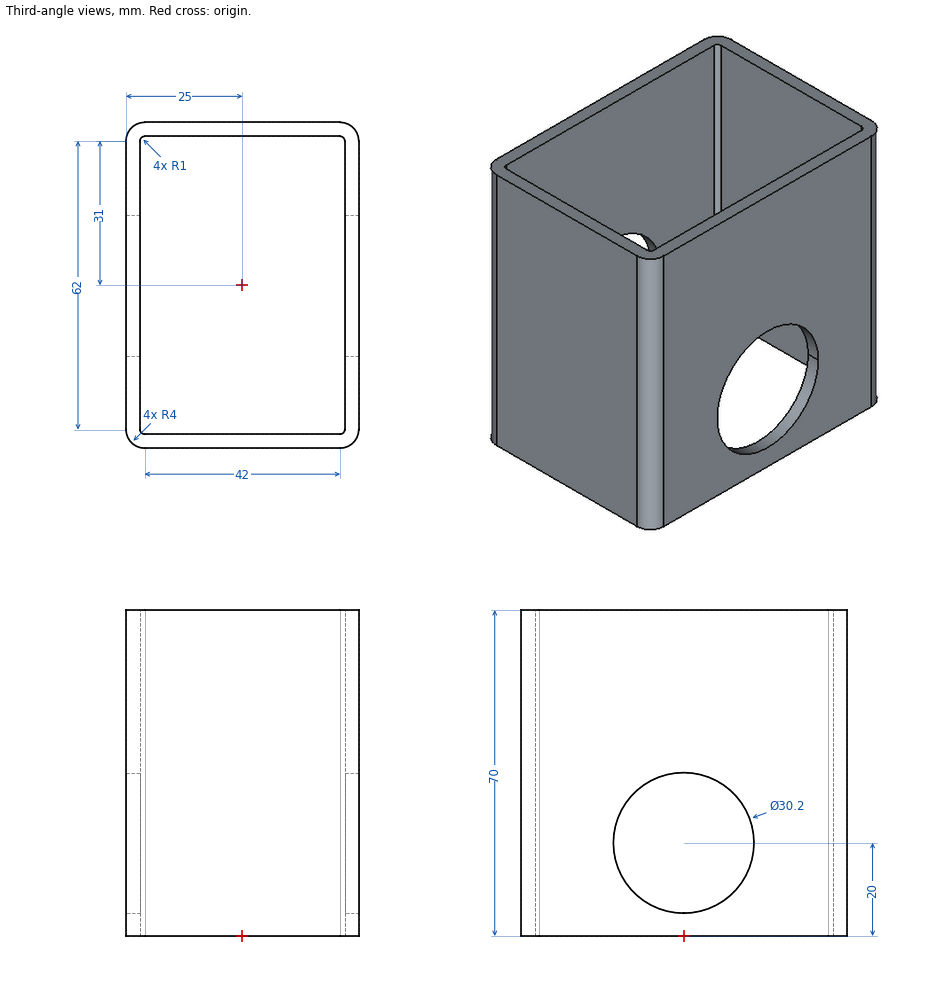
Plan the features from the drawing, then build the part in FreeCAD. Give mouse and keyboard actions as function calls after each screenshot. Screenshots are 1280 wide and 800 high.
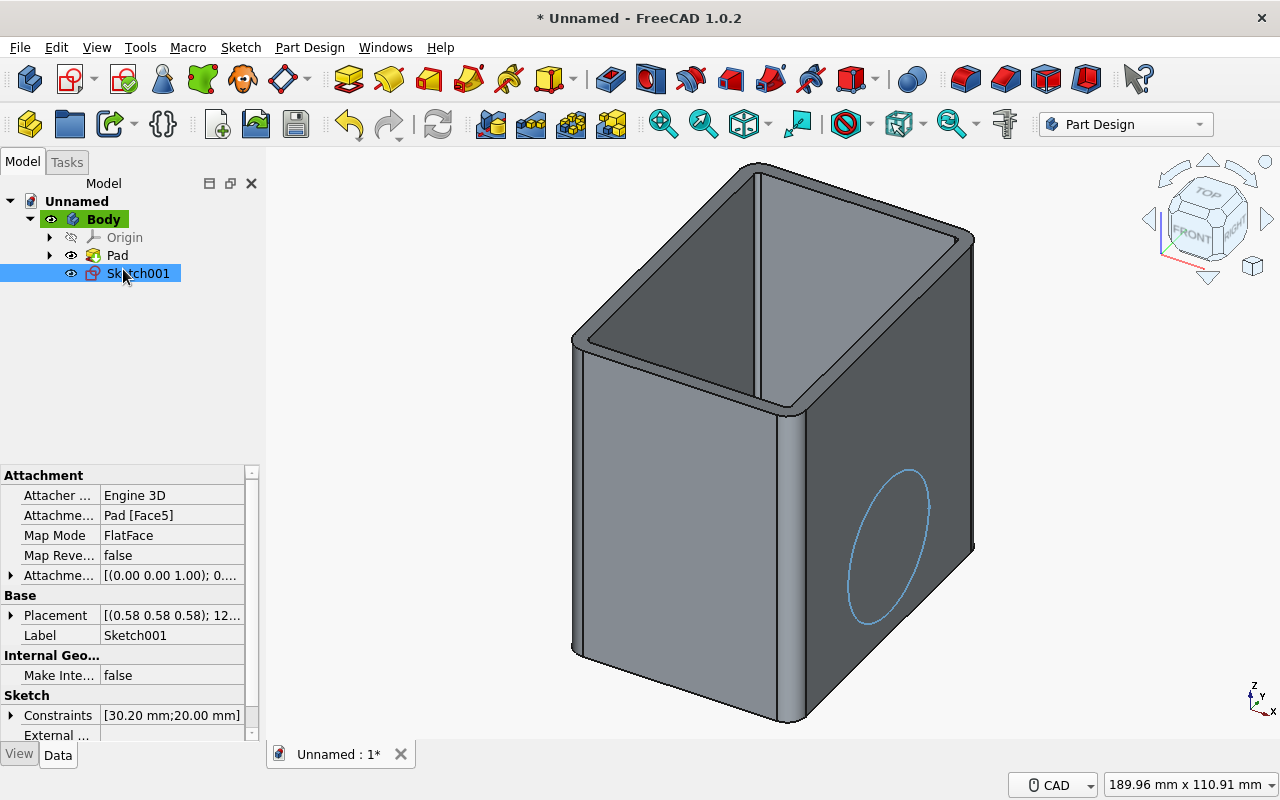
click(612, 80)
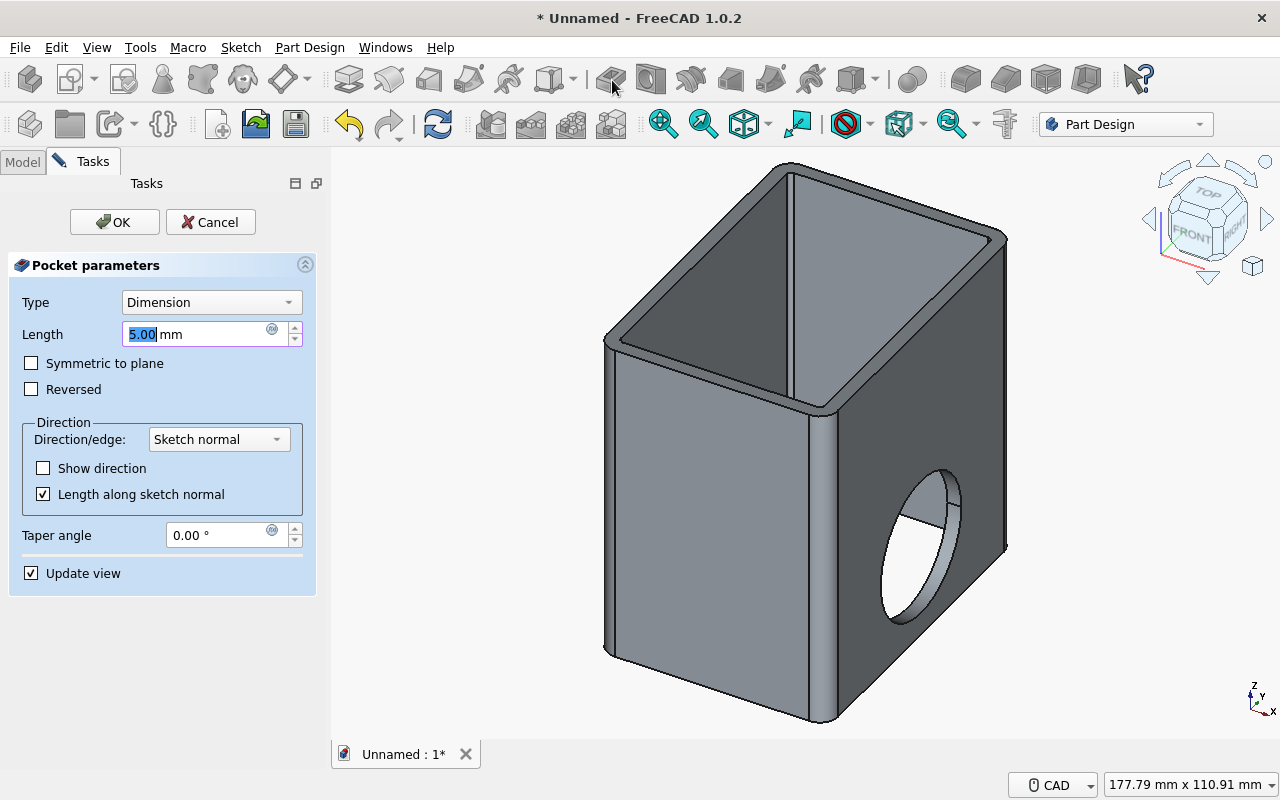
click(212, 302)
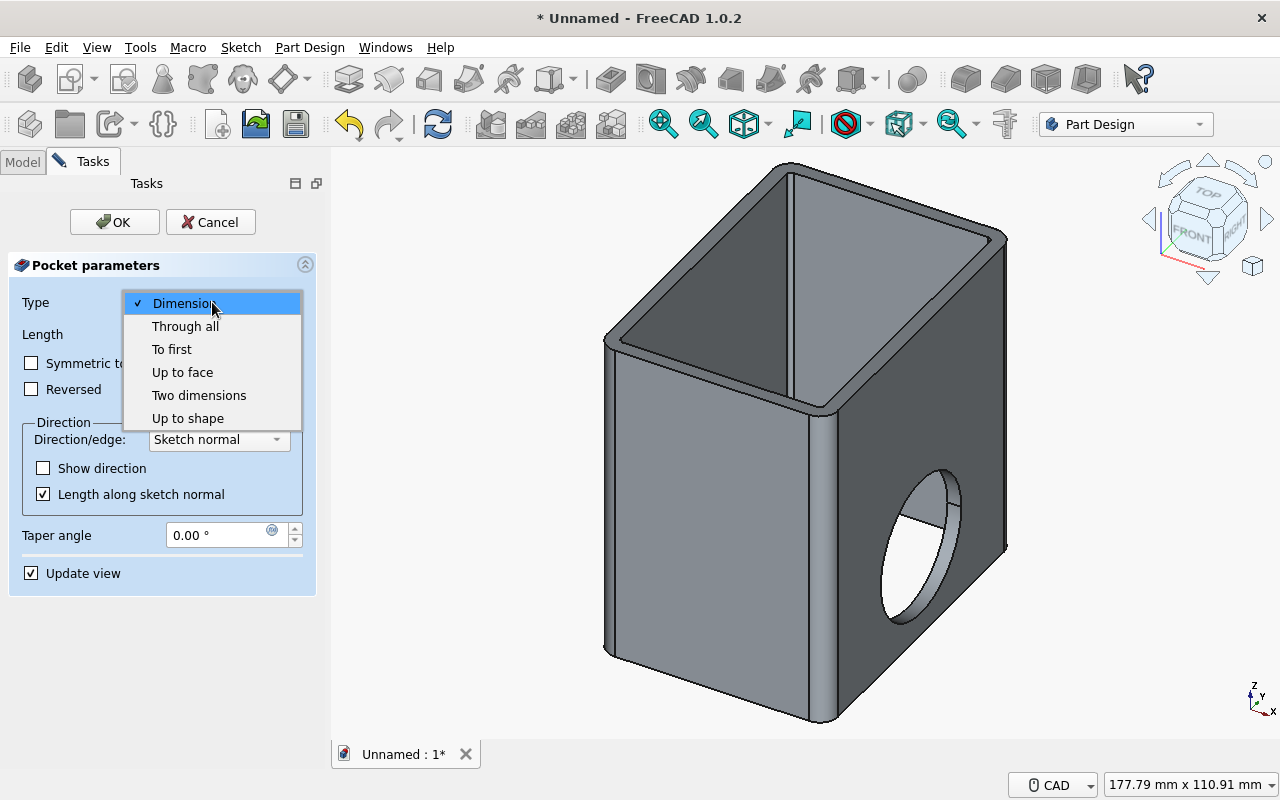
click(212, 326)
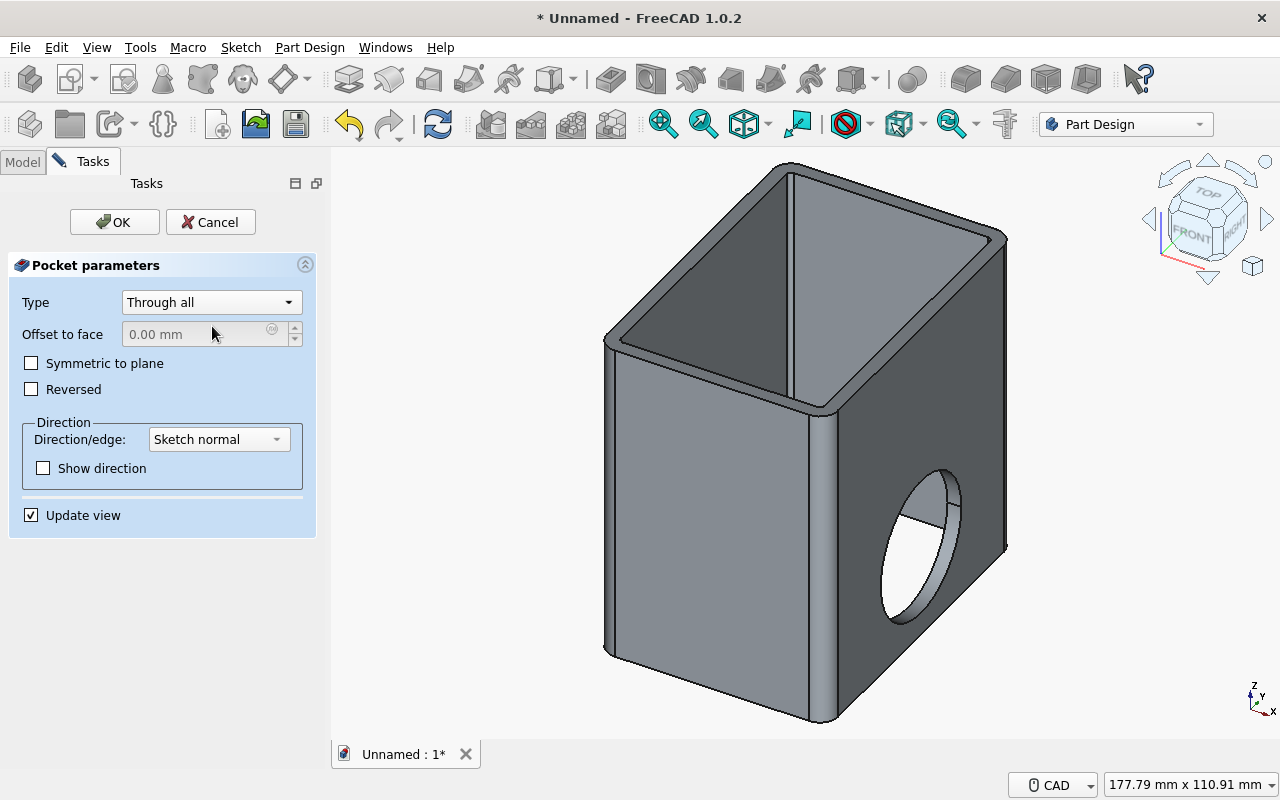
click(115, 222)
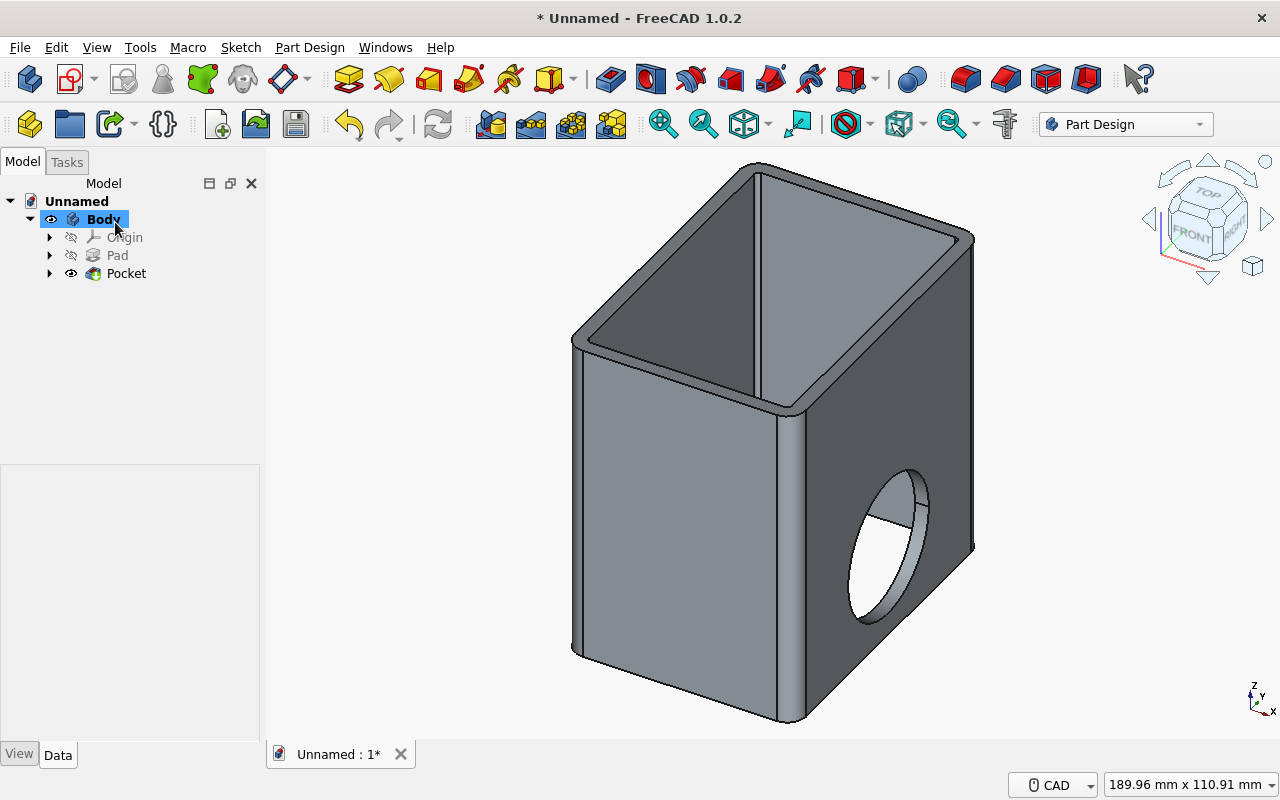
key(0)